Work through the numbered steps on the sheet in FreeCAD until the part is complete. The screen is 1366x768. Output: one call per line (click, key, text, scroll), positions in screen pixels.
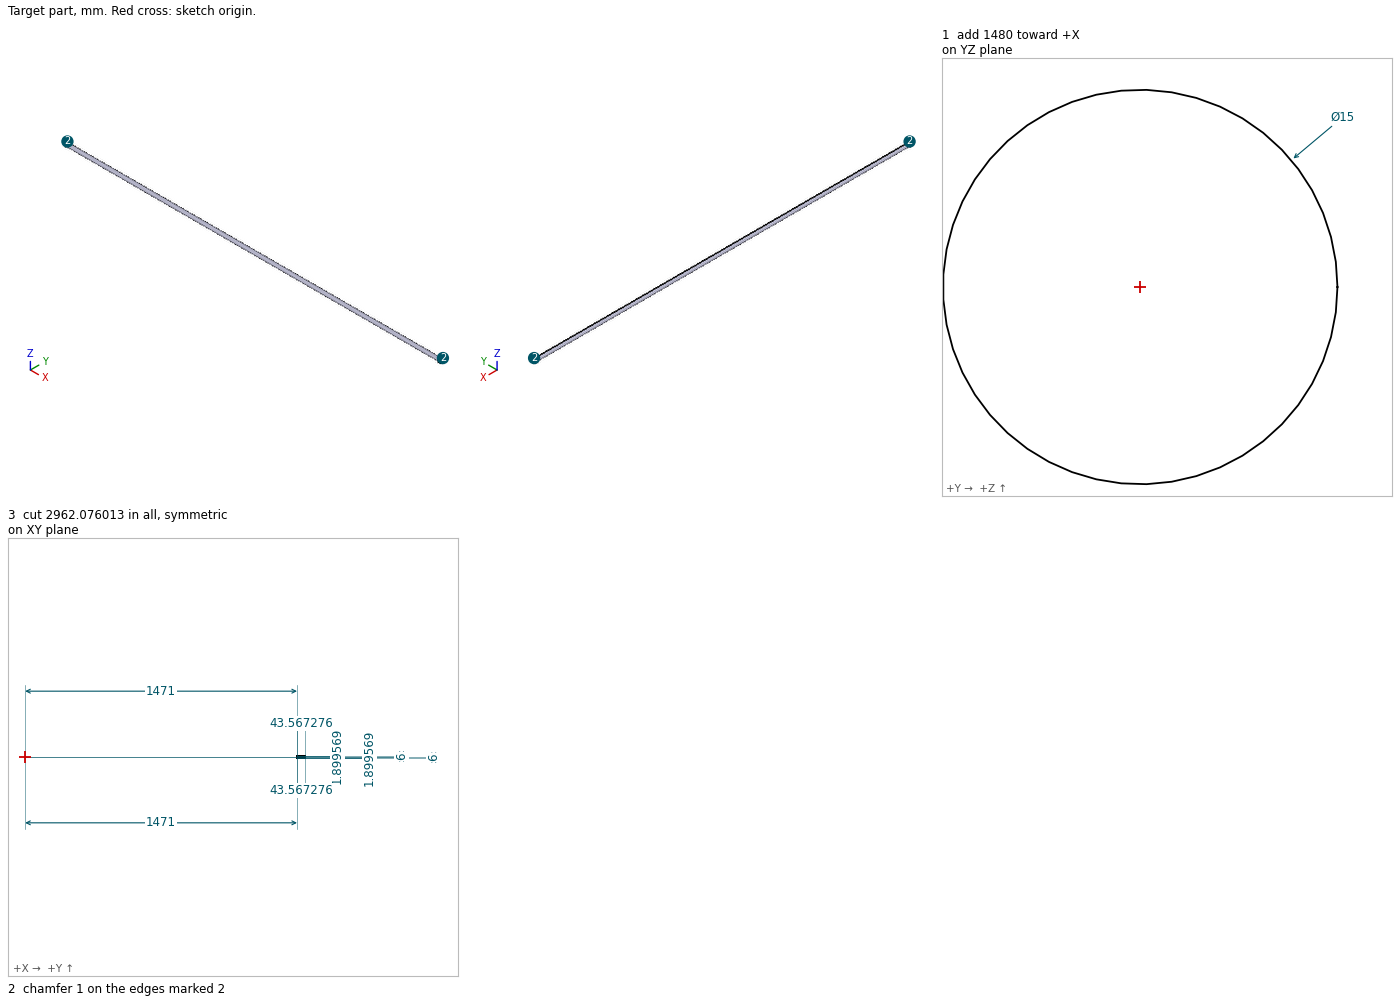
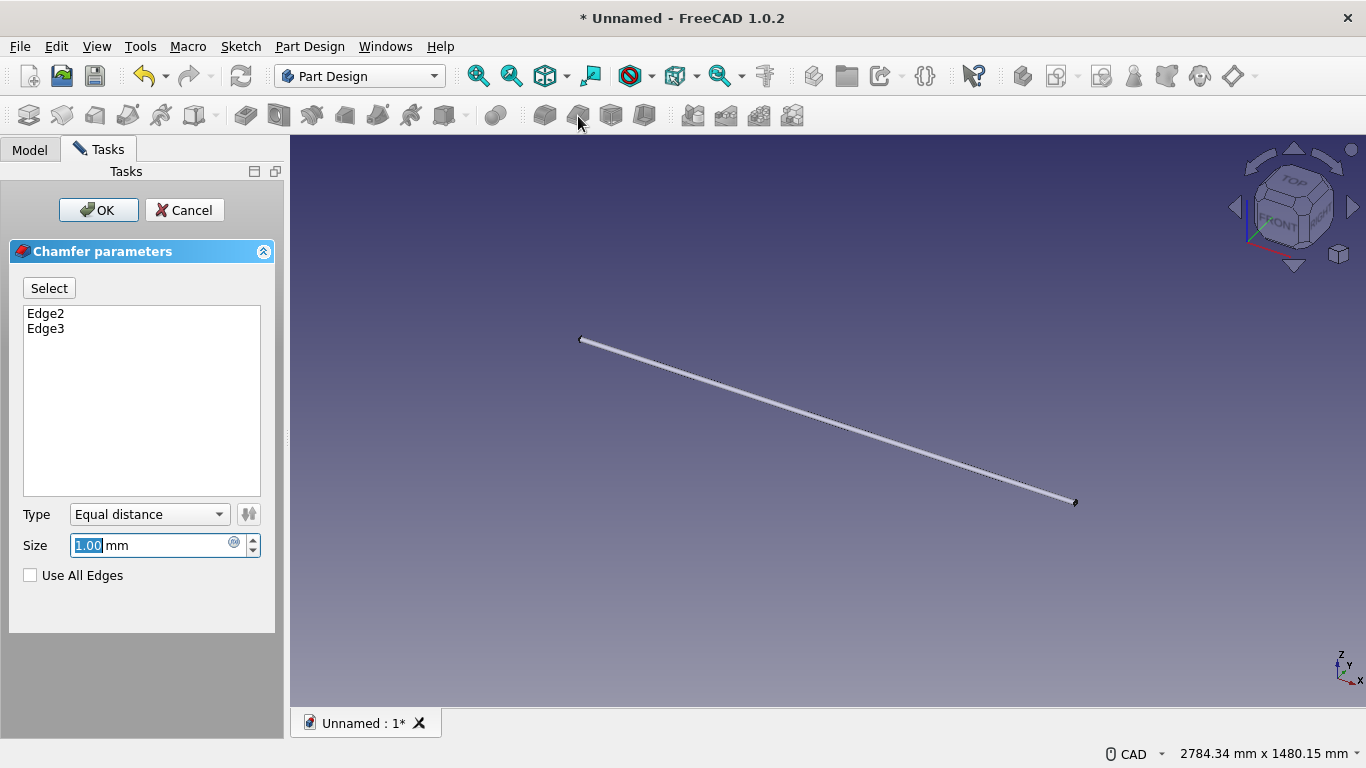
text(1)
key(Tab)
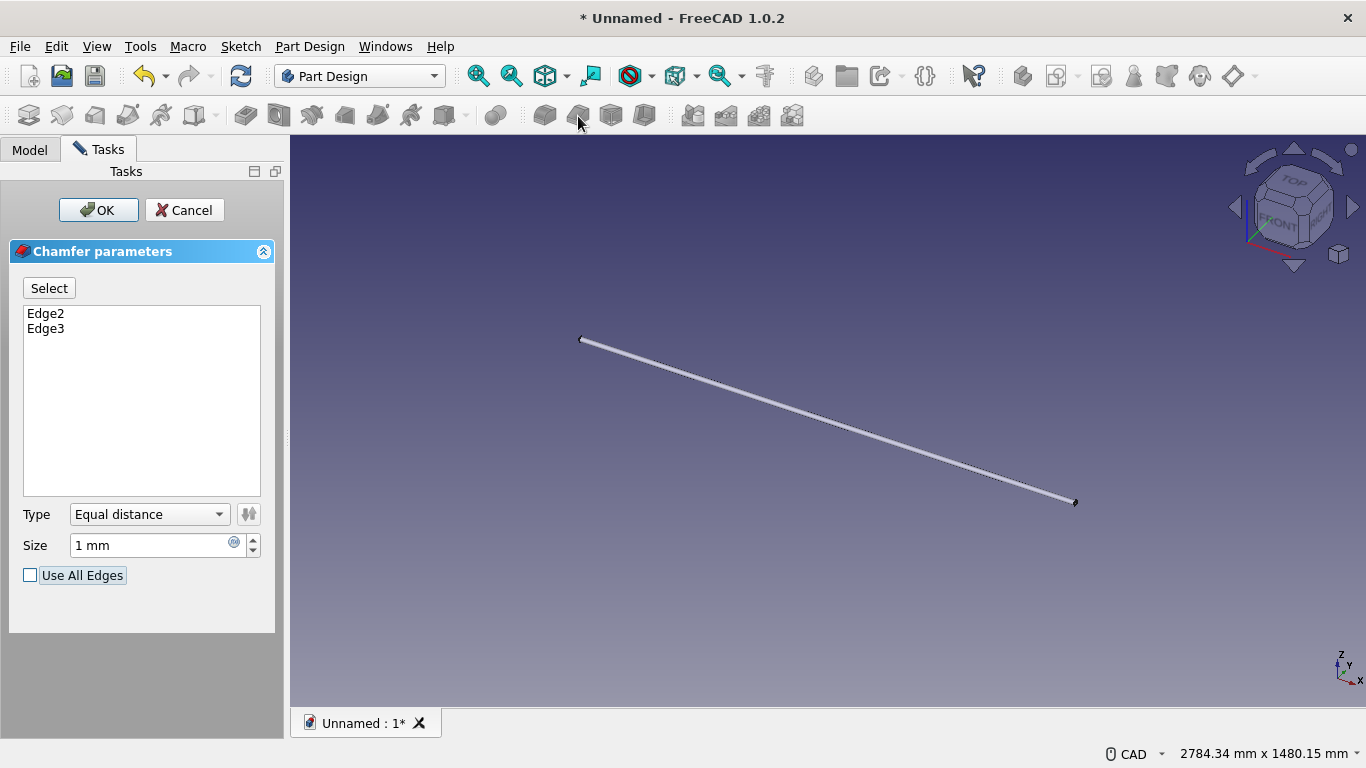
click(99, 210)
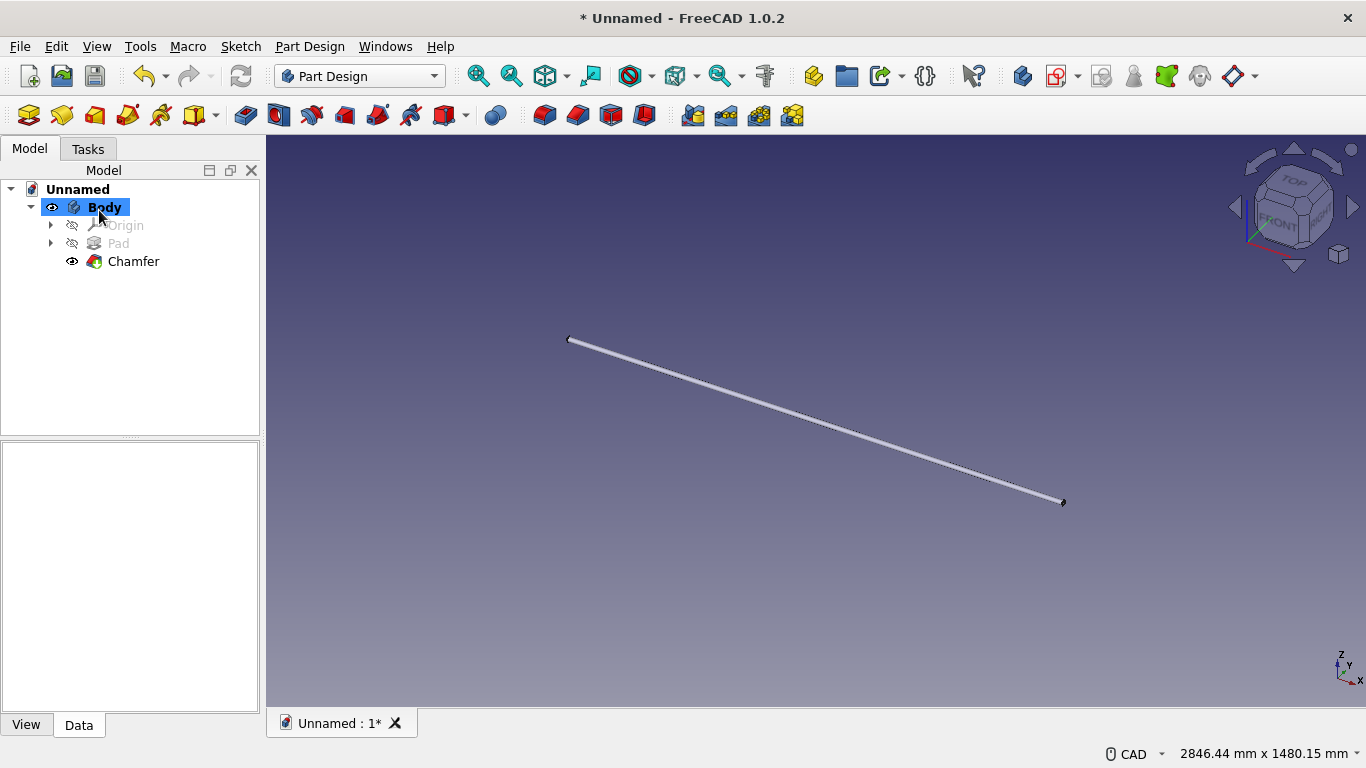
click(1056, 76)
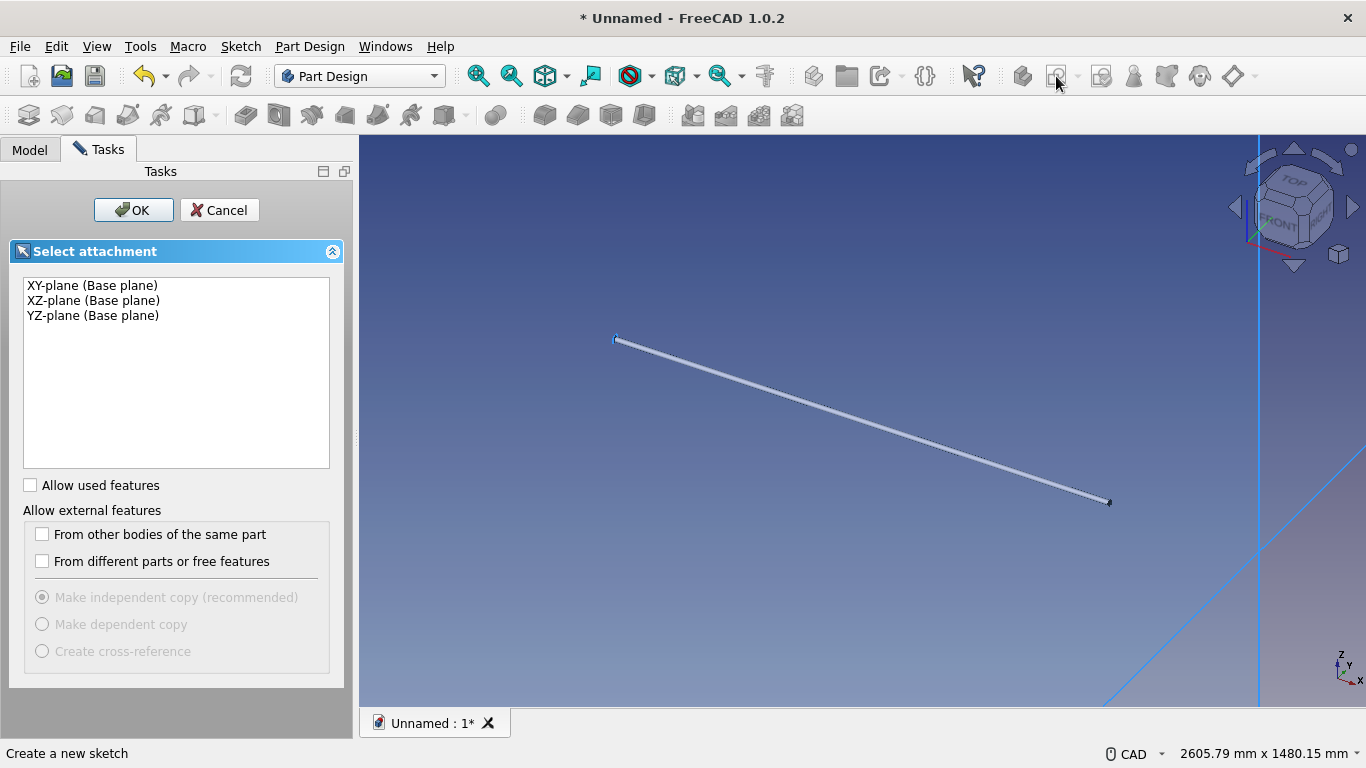
click(84, 286)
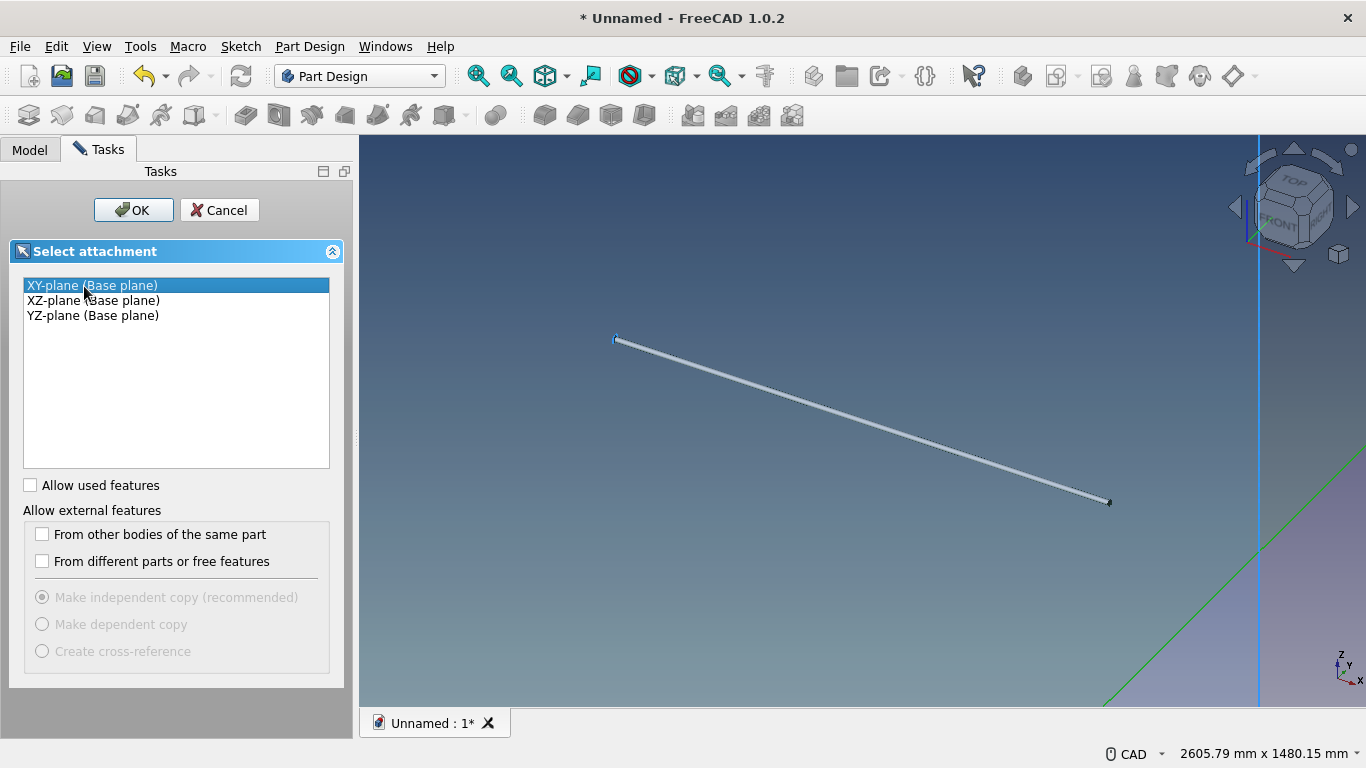
click(134, 210)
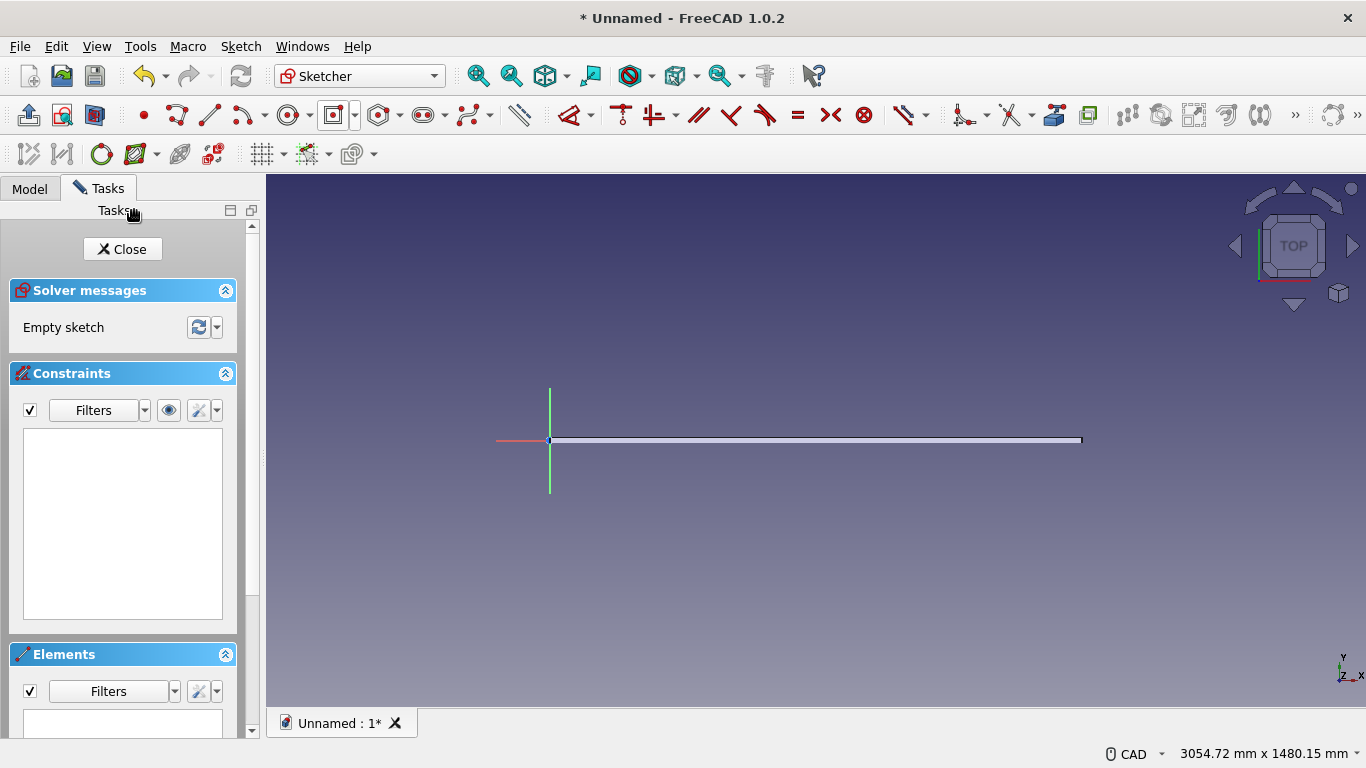
key(q)
key(s)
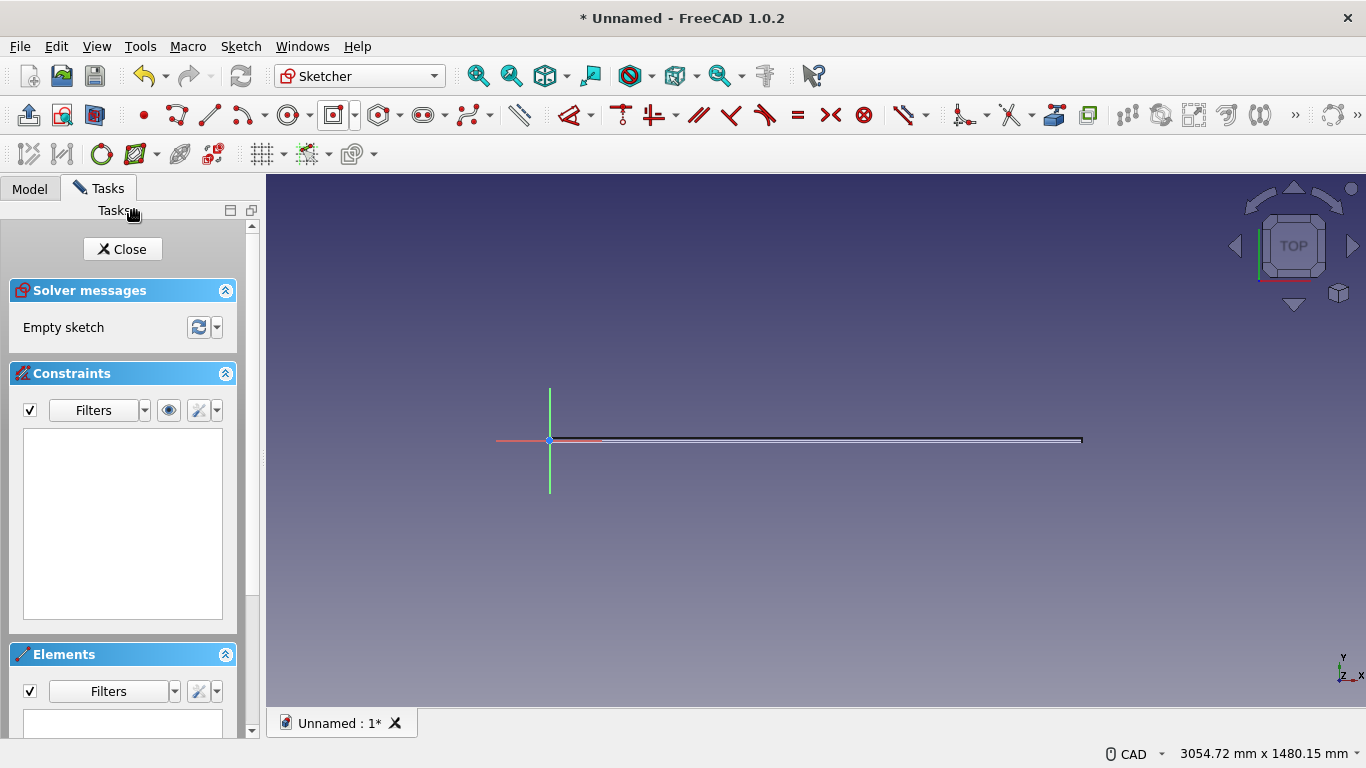
scroll(1105, 440, up, 15)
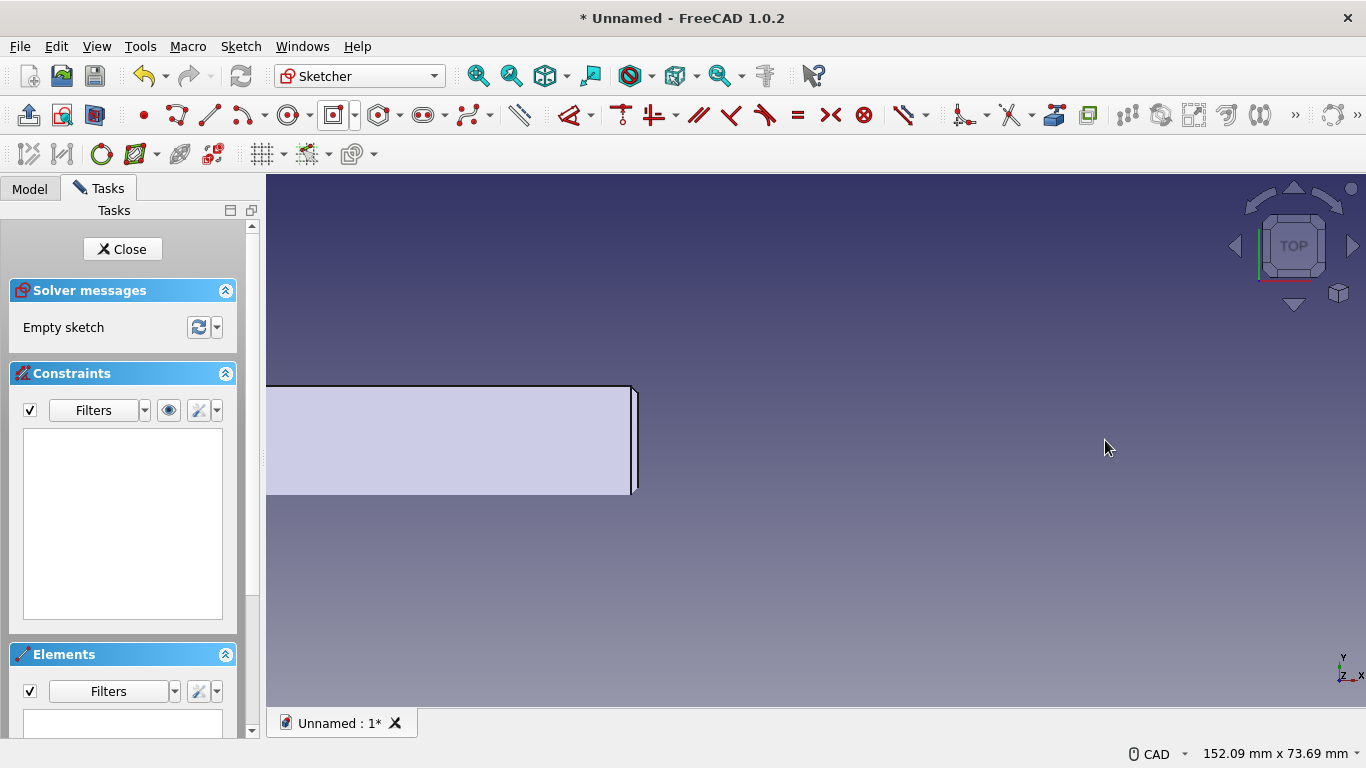
scroll(716, 440, up, 4)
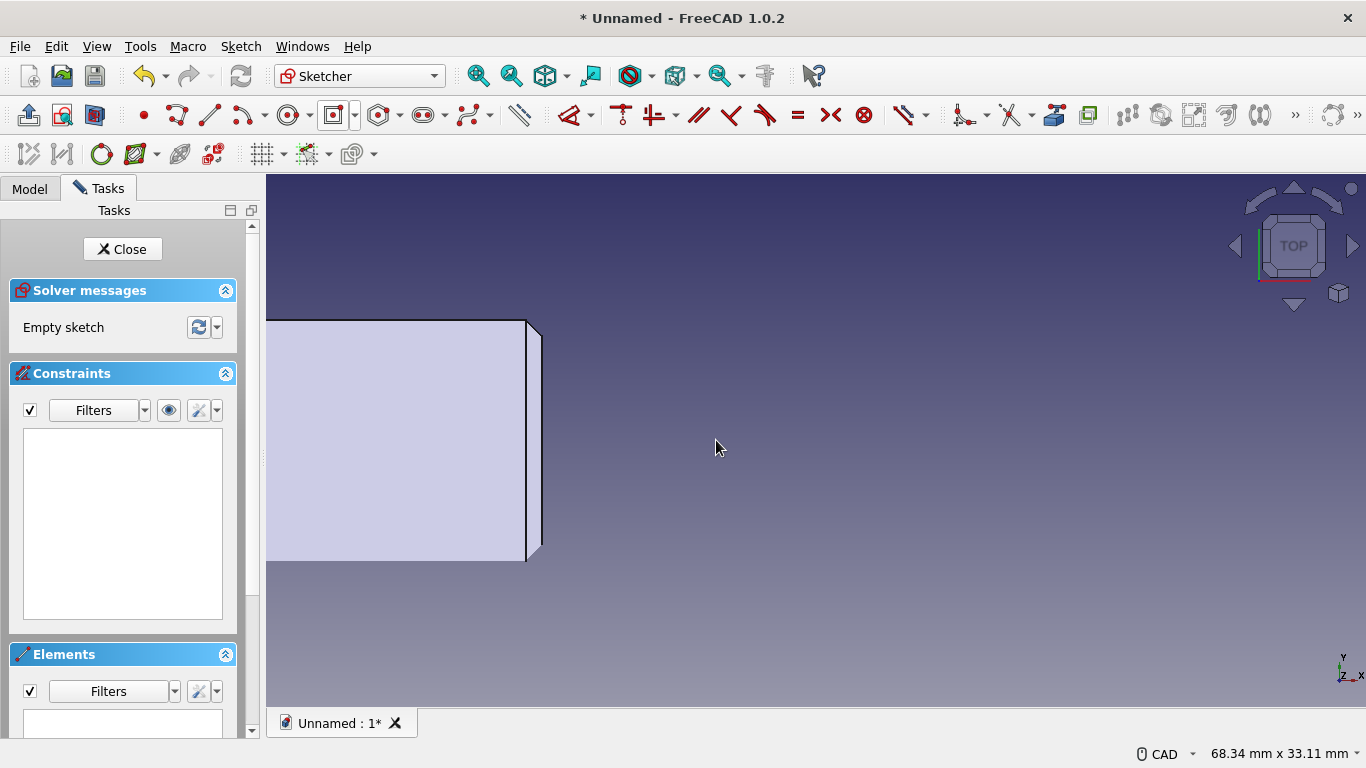
key(g)
key(r)